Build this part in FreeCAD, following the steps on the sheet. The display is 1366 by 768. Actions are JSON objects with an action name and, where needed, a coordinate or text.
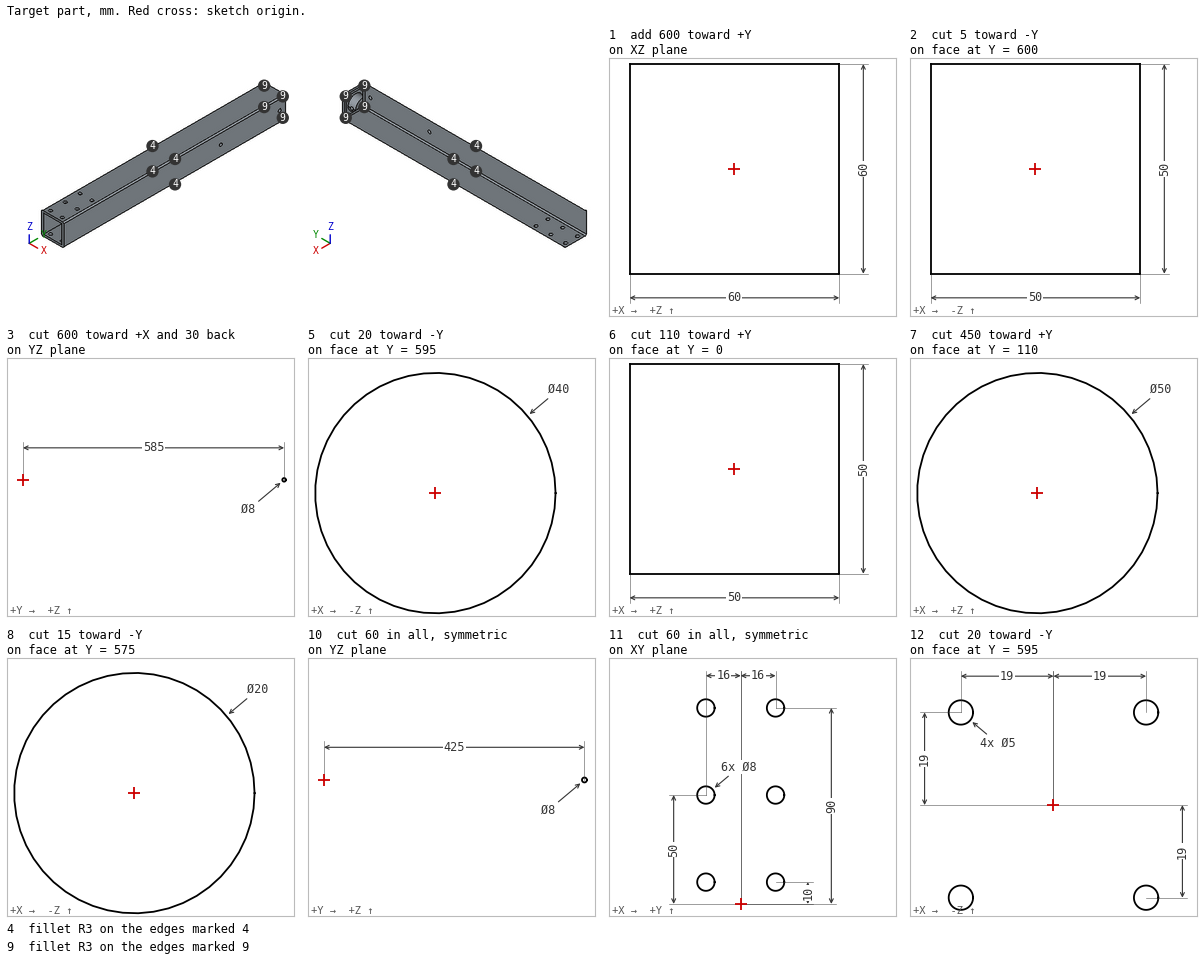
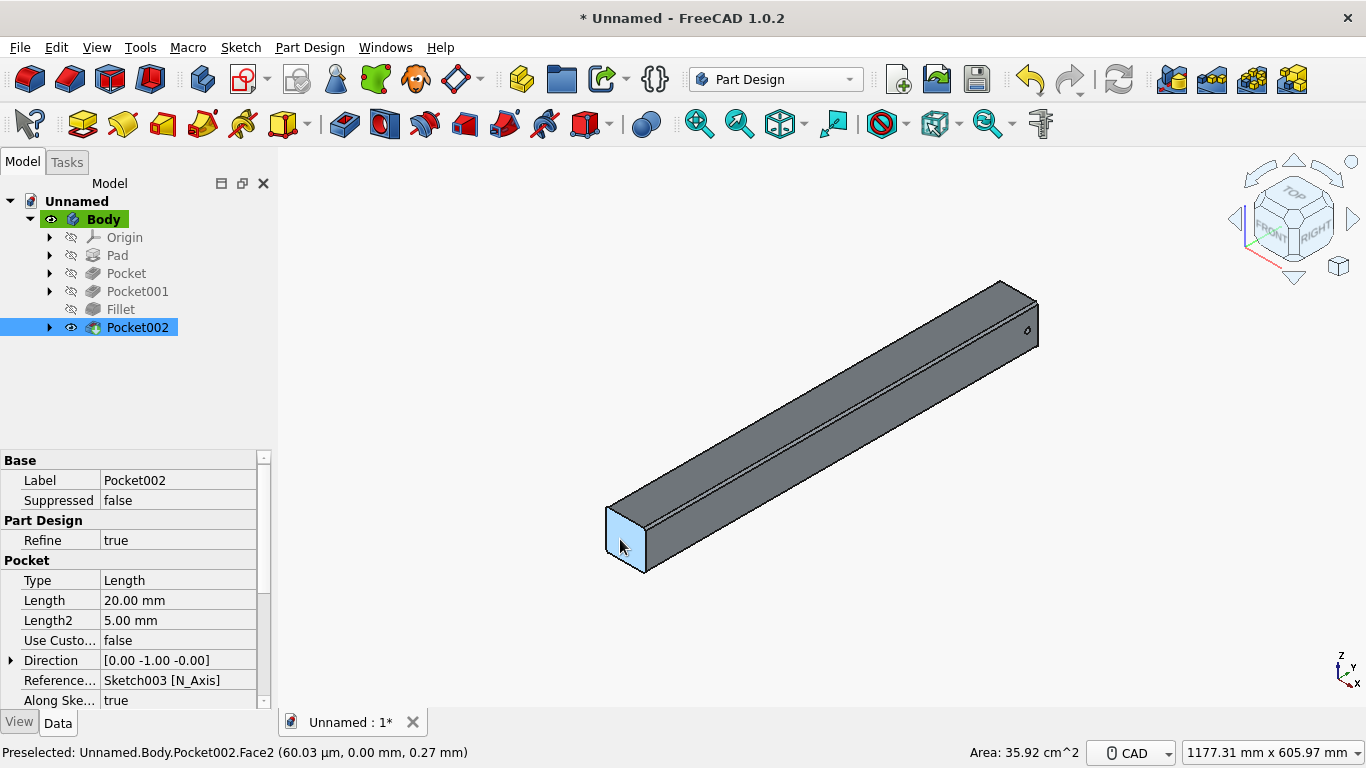
{"action": "left_click", "coordinate": [244, 80]}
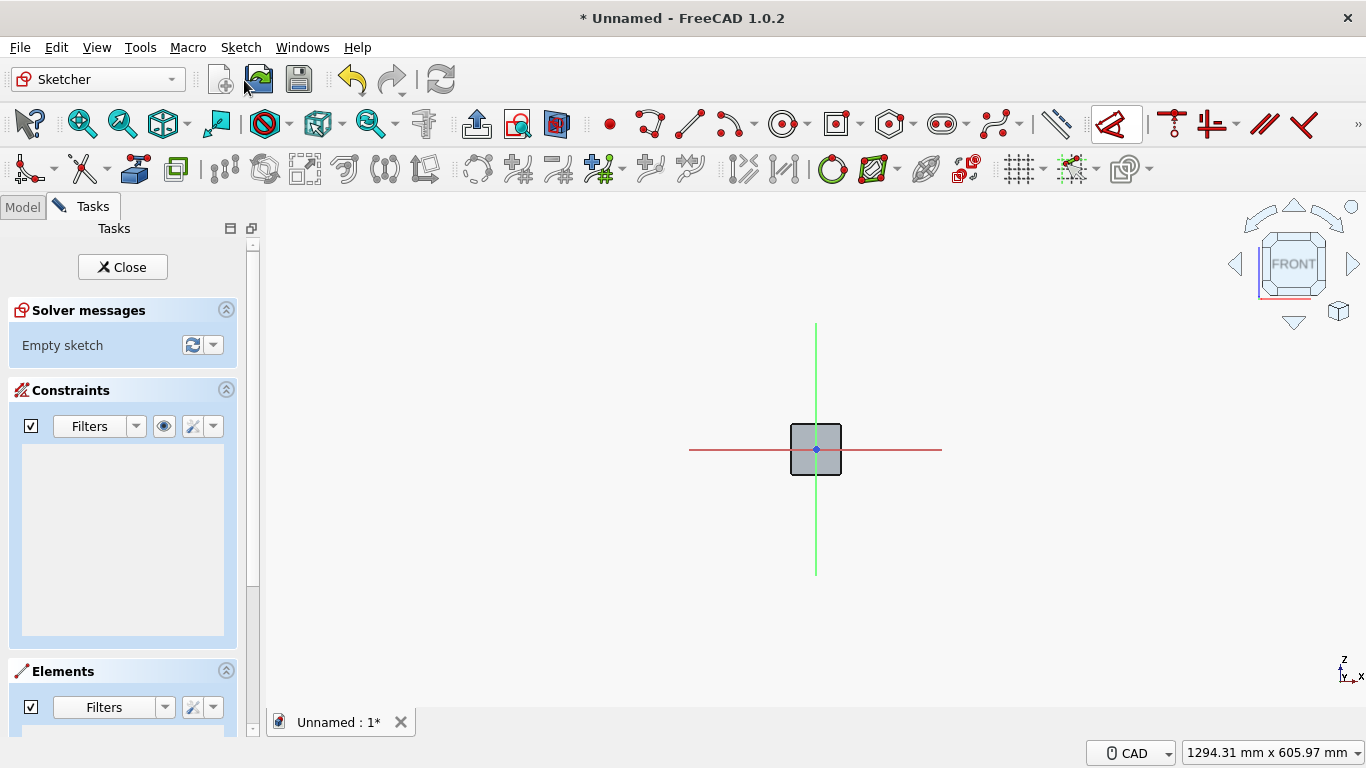
{"action": "scroll", "coordinate": [827, 450], "scroll_direction": "up", "scroll_amount": 10}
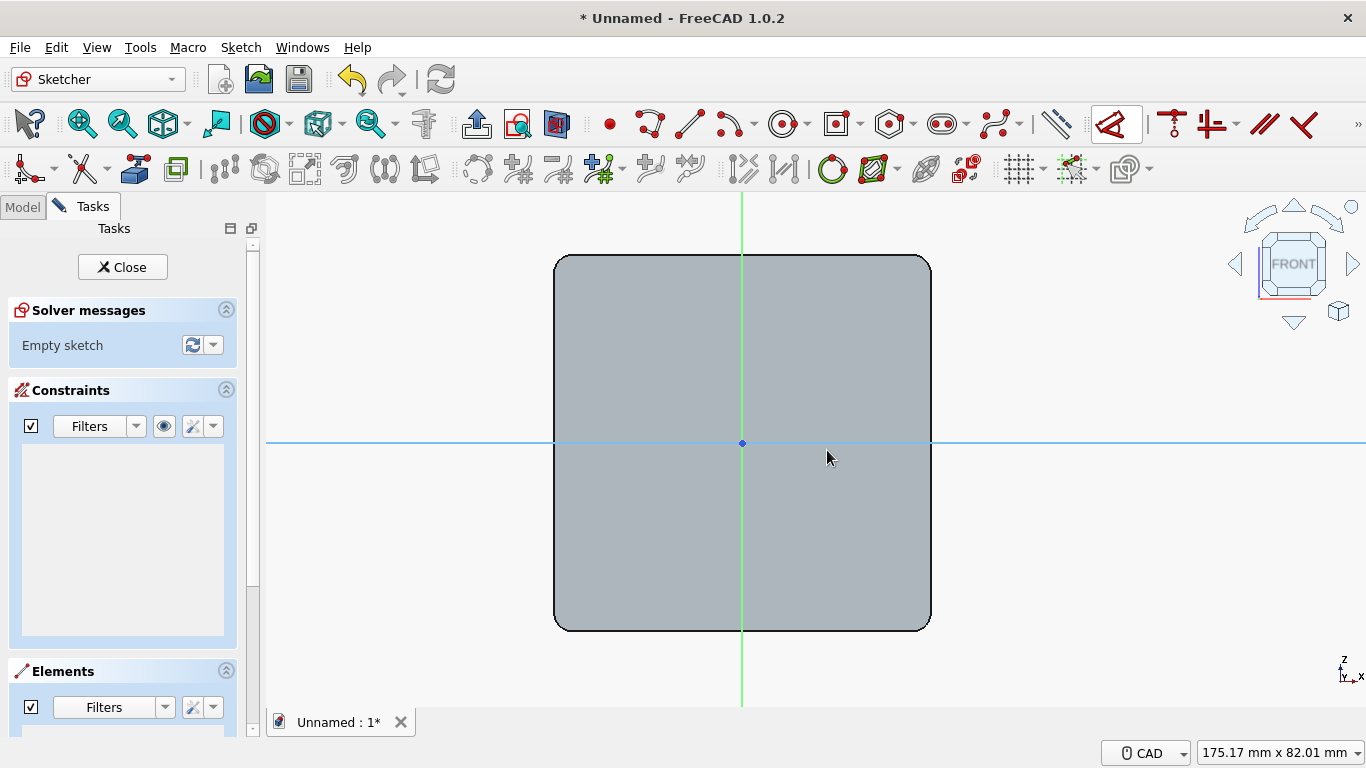
{"action": "left_click", "coordinate": [836, 124]}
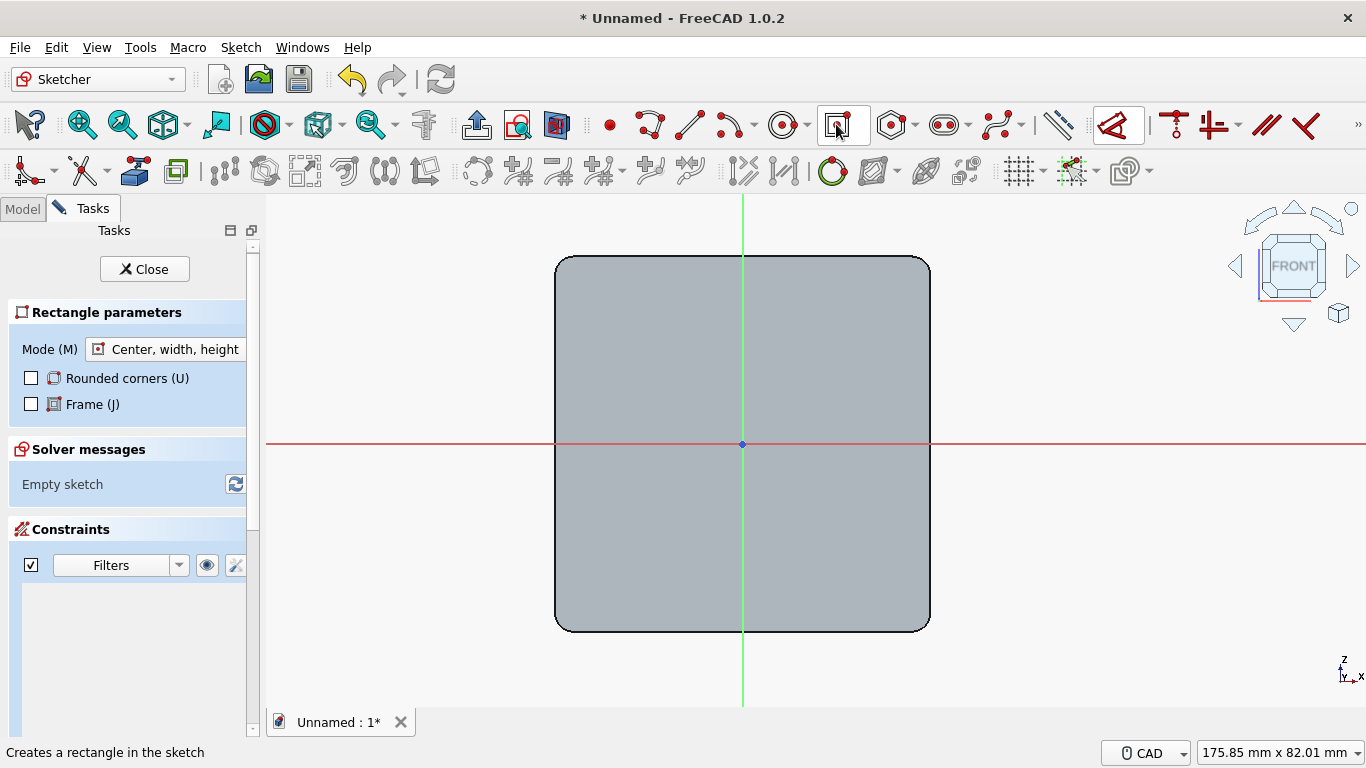
{"action": "left_click", "coordinate": [743, 444]}
{"action": "mouse_move", "coordinate": [899, 288]}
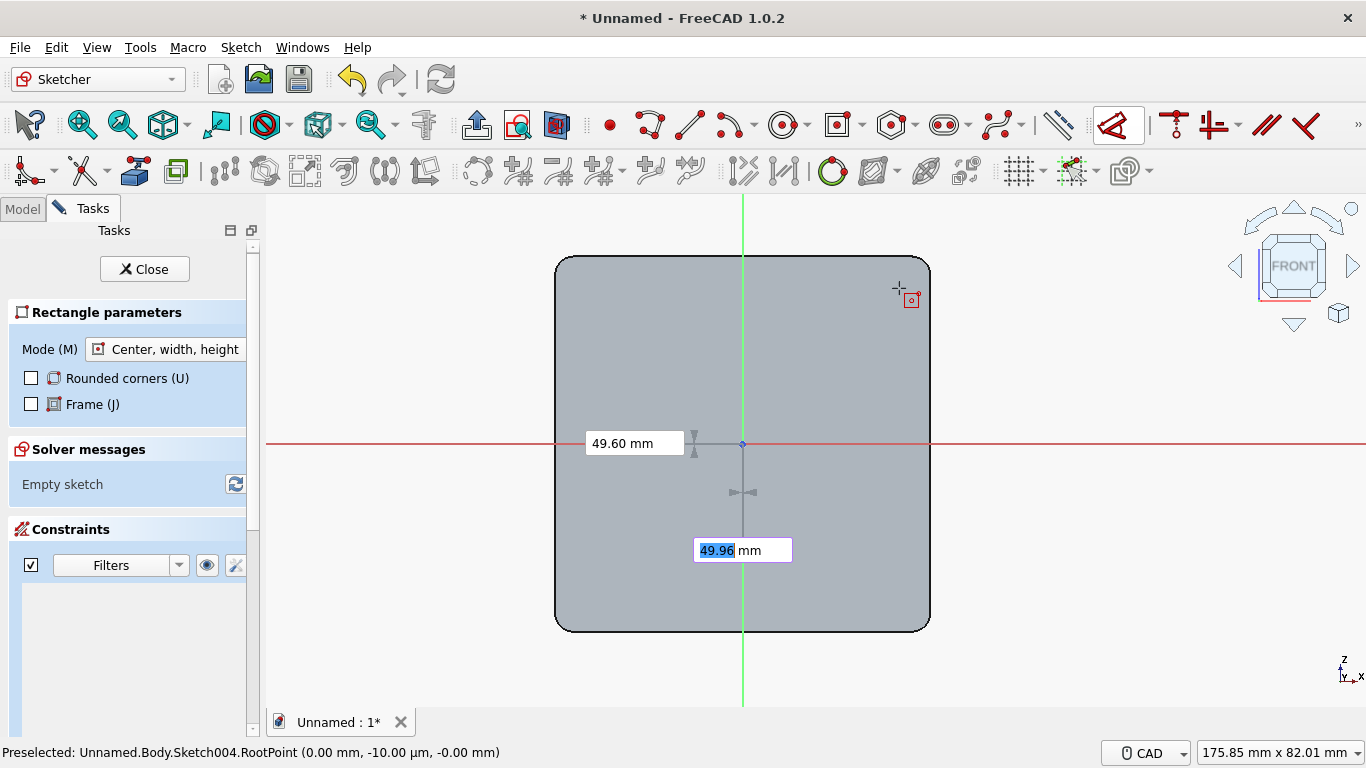
{"action": "type", "text": "50"}
{"action": "key", "text": "Tab"}
{"action": "type", "text": "50"}
{"action": "key", "text": "Return"}
{"action": "key", "text": "Escape"}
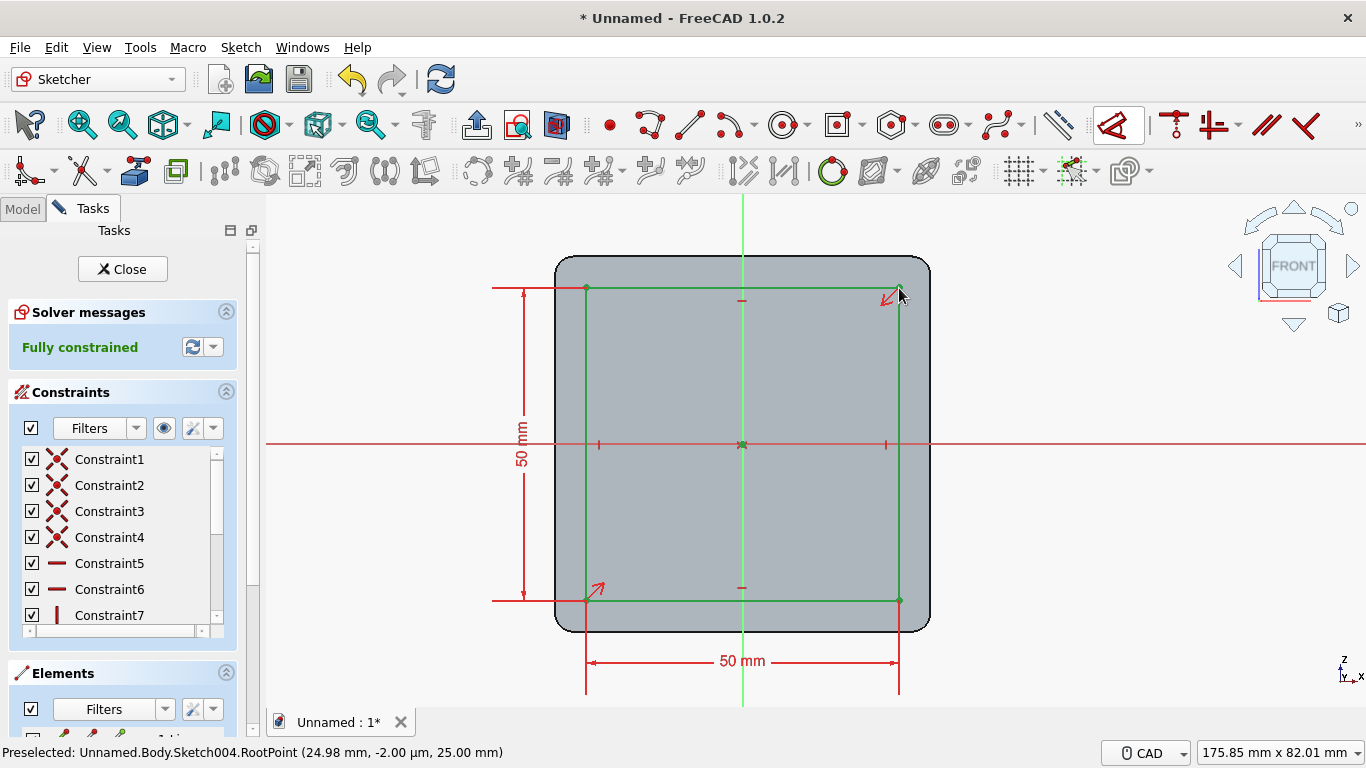
{"action": "left_click", "coordinate": [123, 269]}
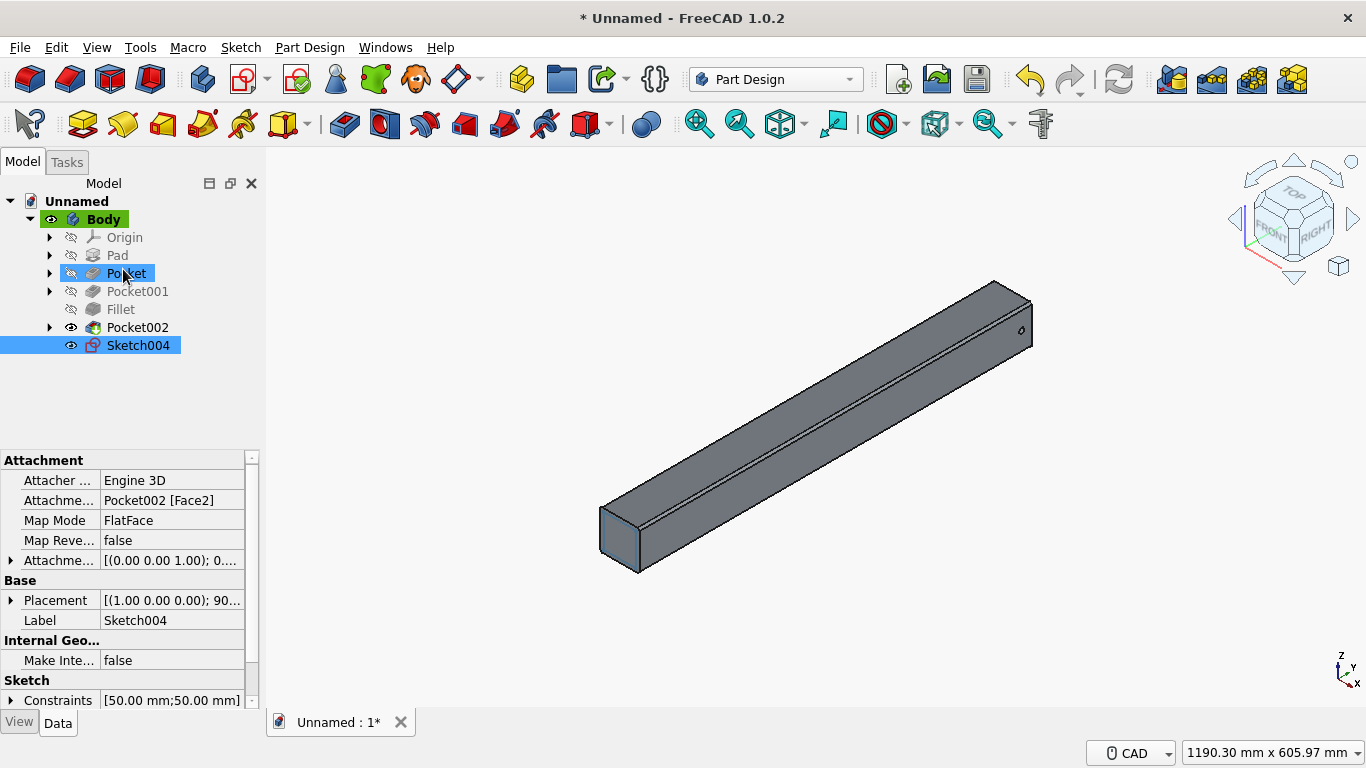
{"action": "left_click", "coordinate": [346, 124]}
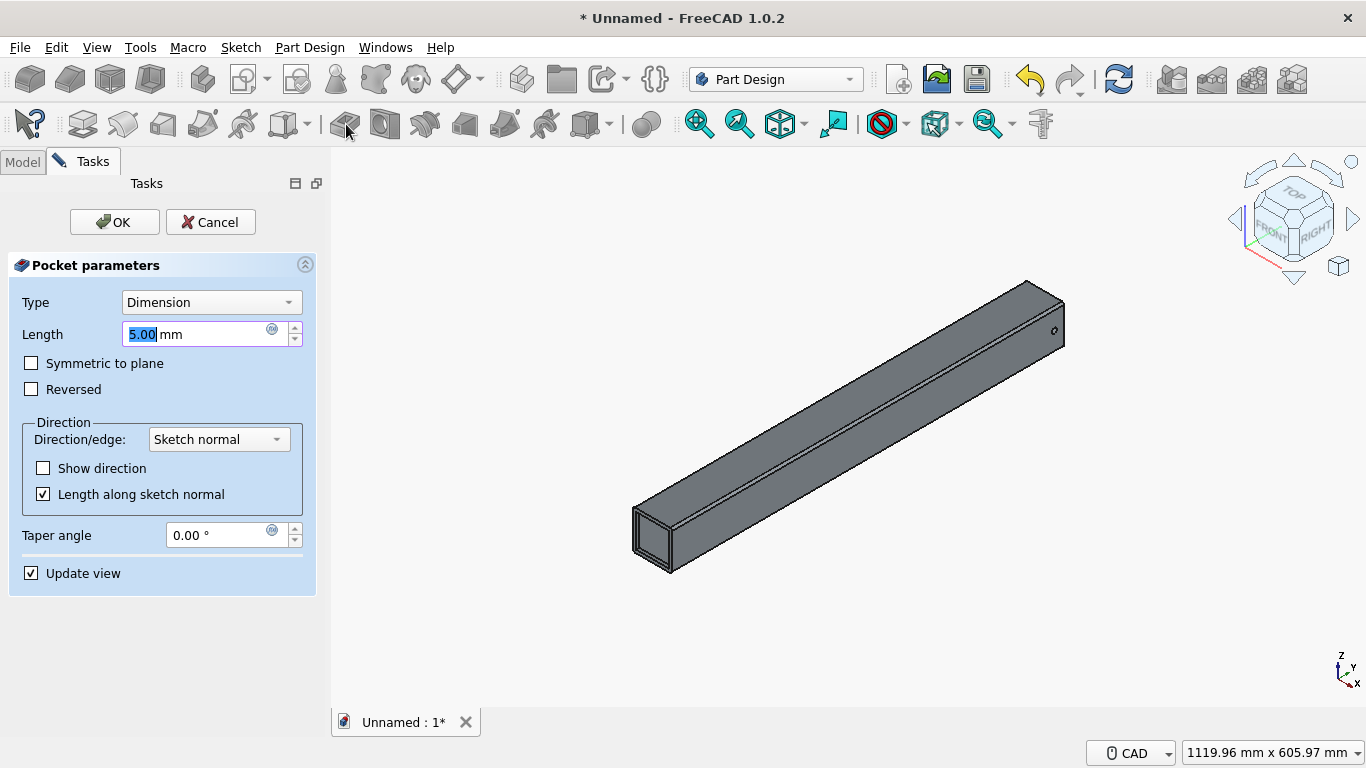
{"action": "type", "text": "110"}
{"action": "key", "text": "Tab"}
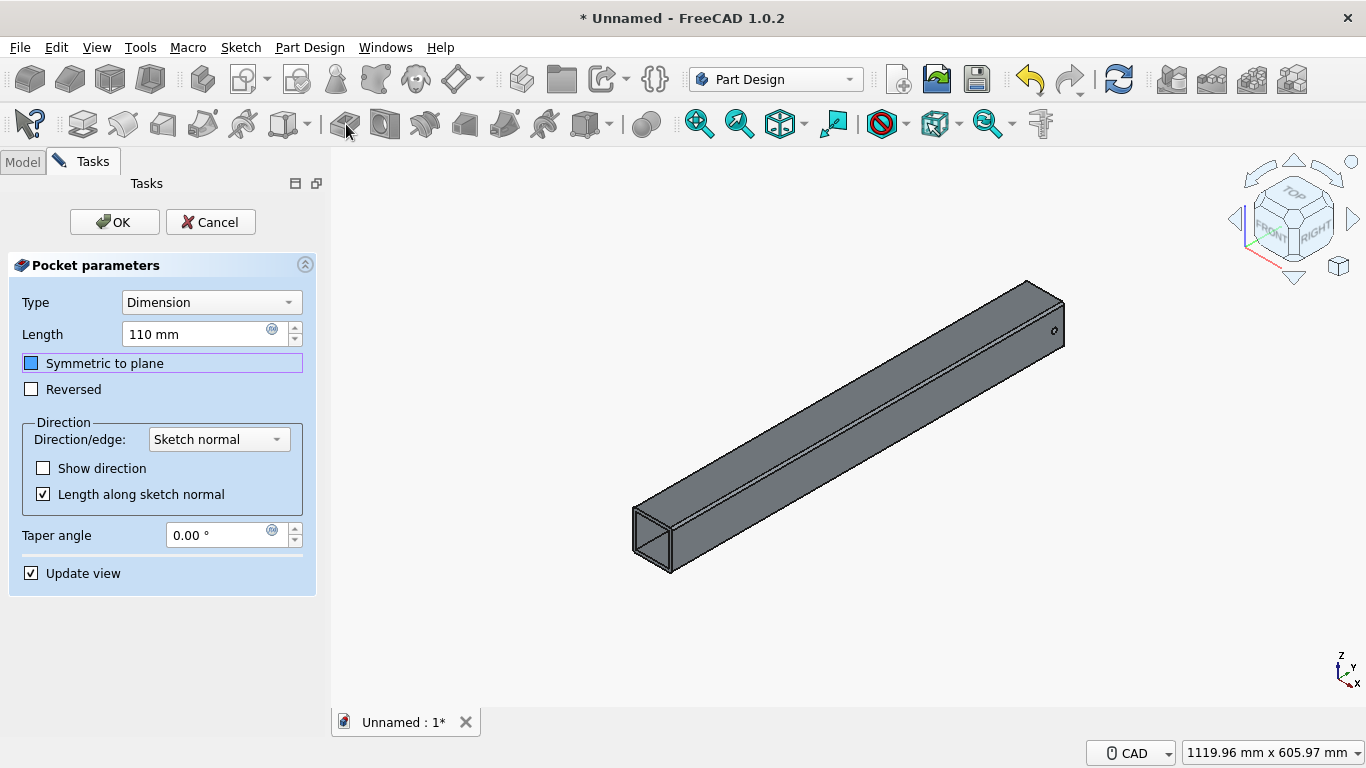
{"action": "left_click", "coordinate": [115, 222]}